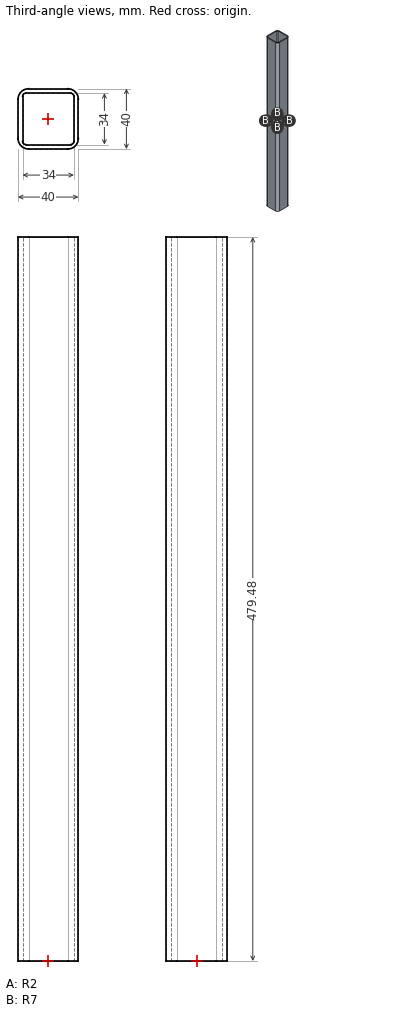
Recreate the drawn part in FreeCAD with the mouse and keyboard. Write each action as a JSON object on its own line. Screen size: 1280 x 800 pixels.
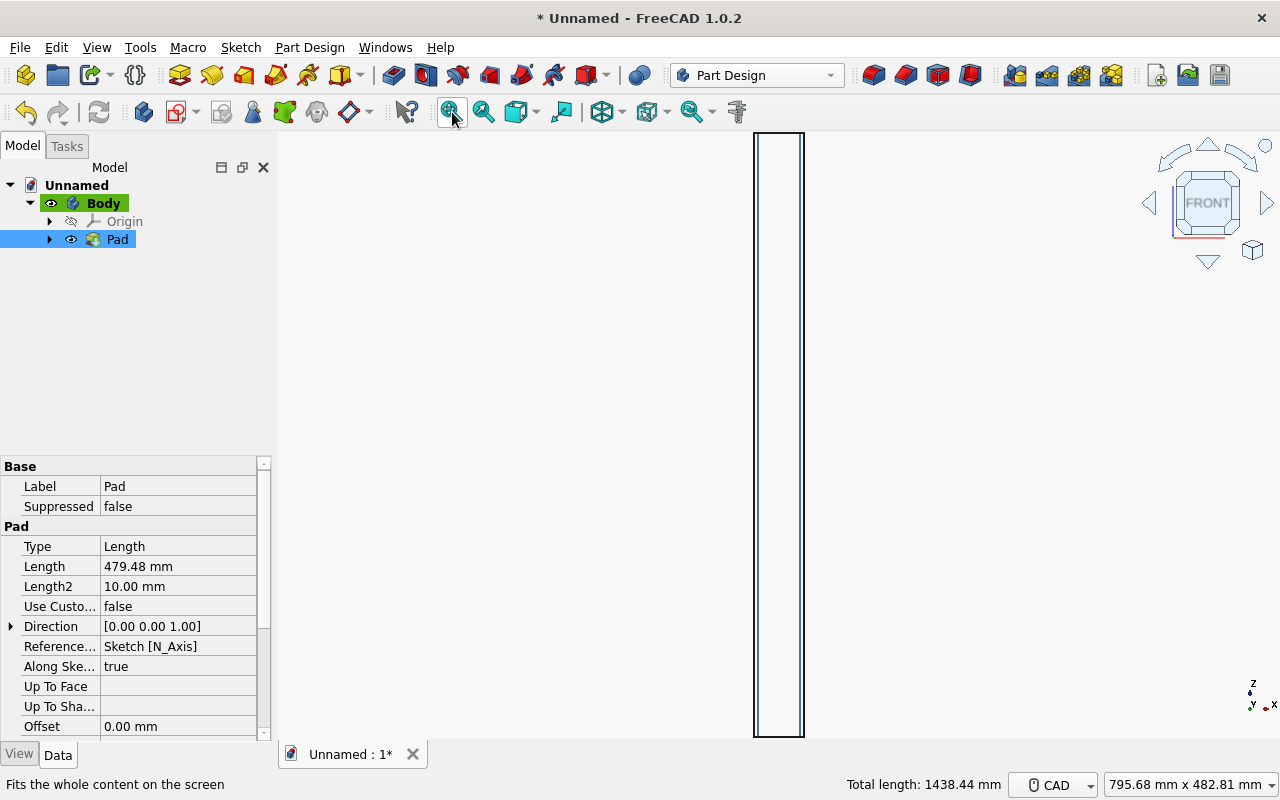
{"action": "key", "text": "3"}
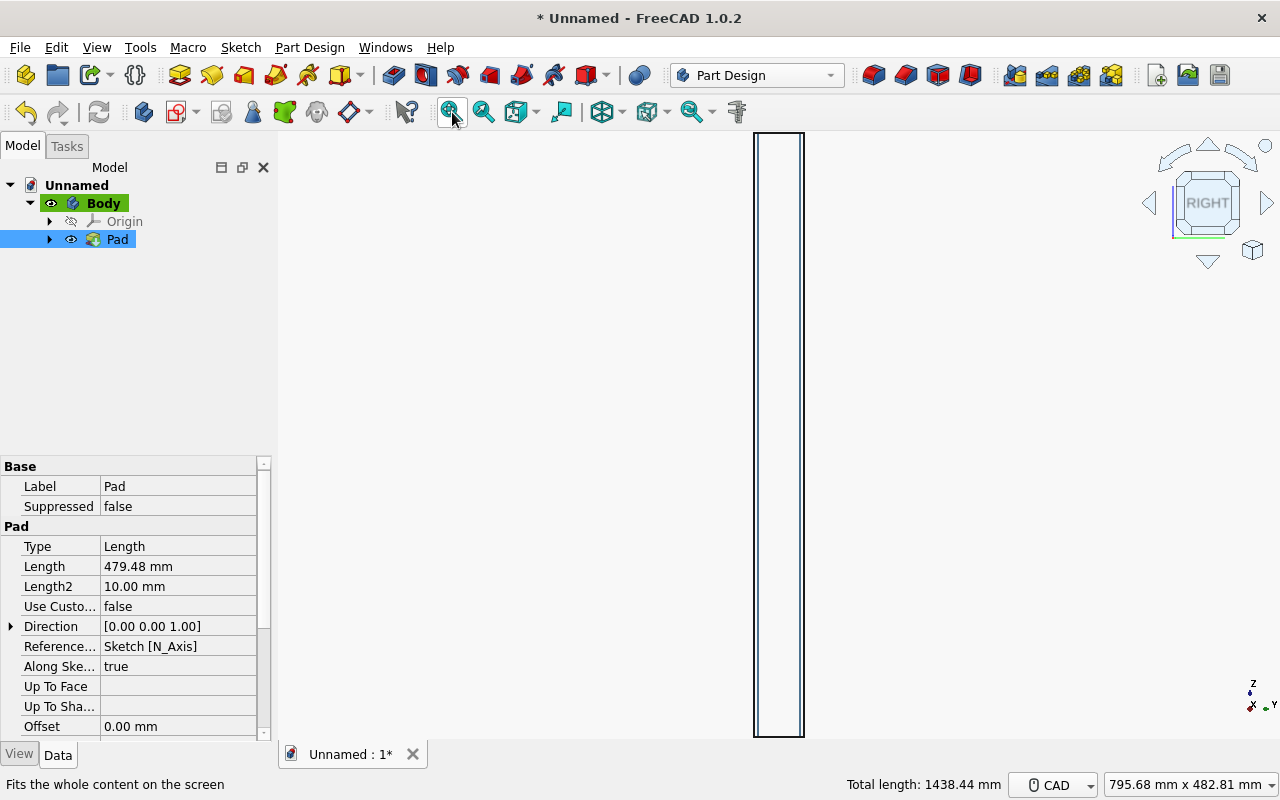
{"action": "scroll", "coordinate": [800, 434], "scroll_direction": "up", "scroll_amount": 6}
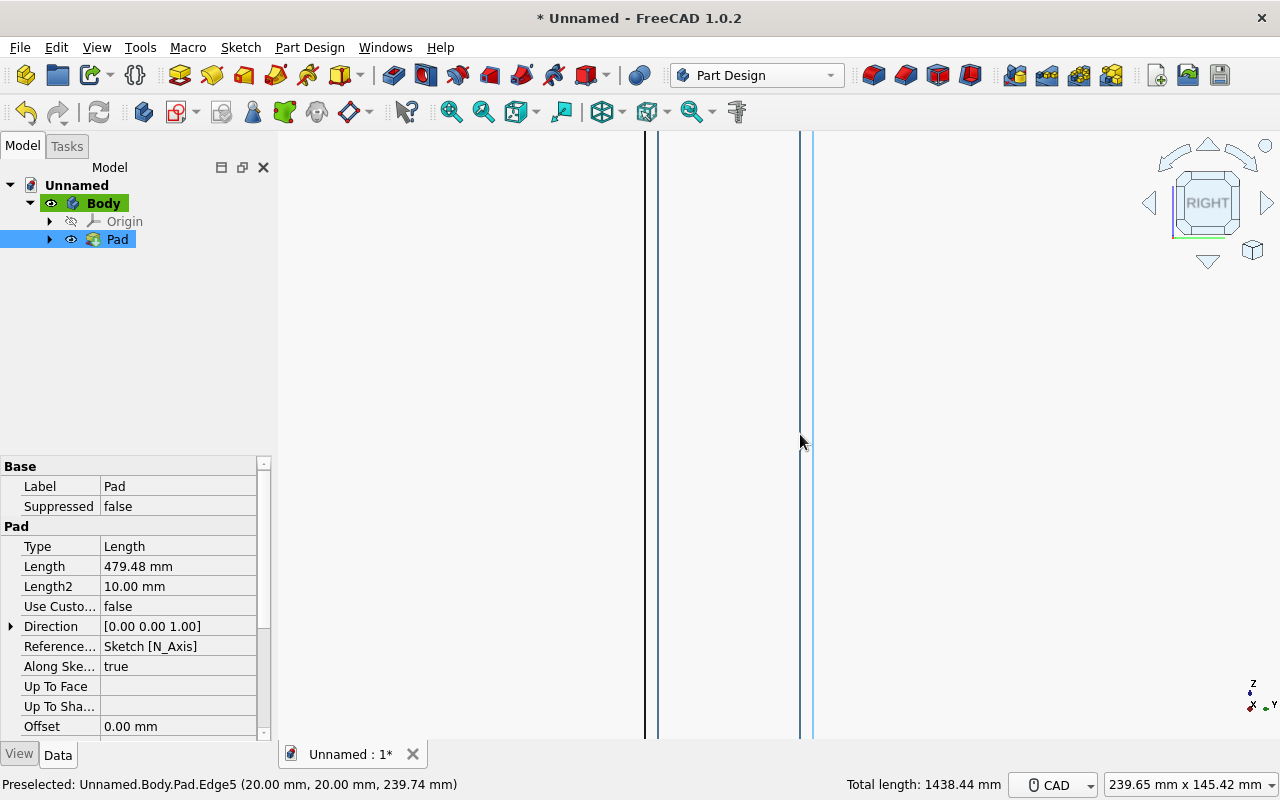
{"action": "key", "text": "v f"}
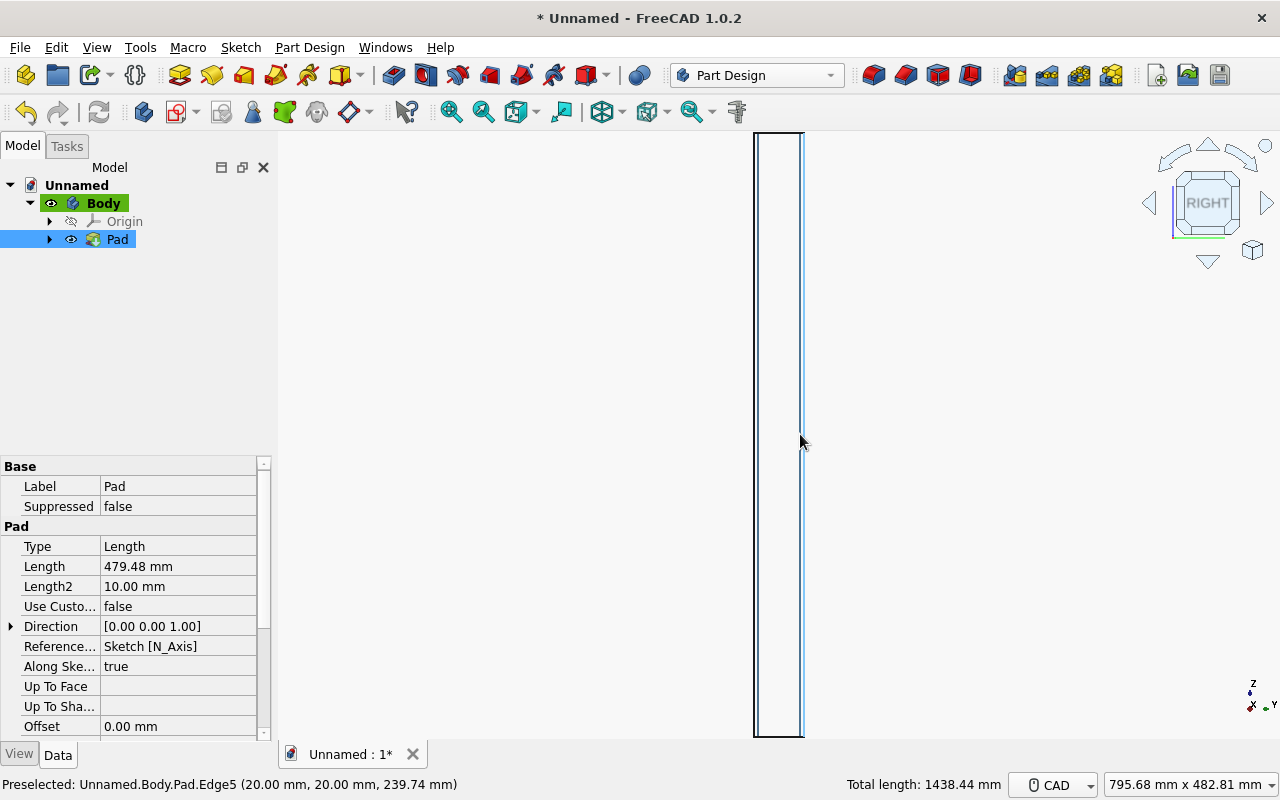
{"action": "key", "text": "5"}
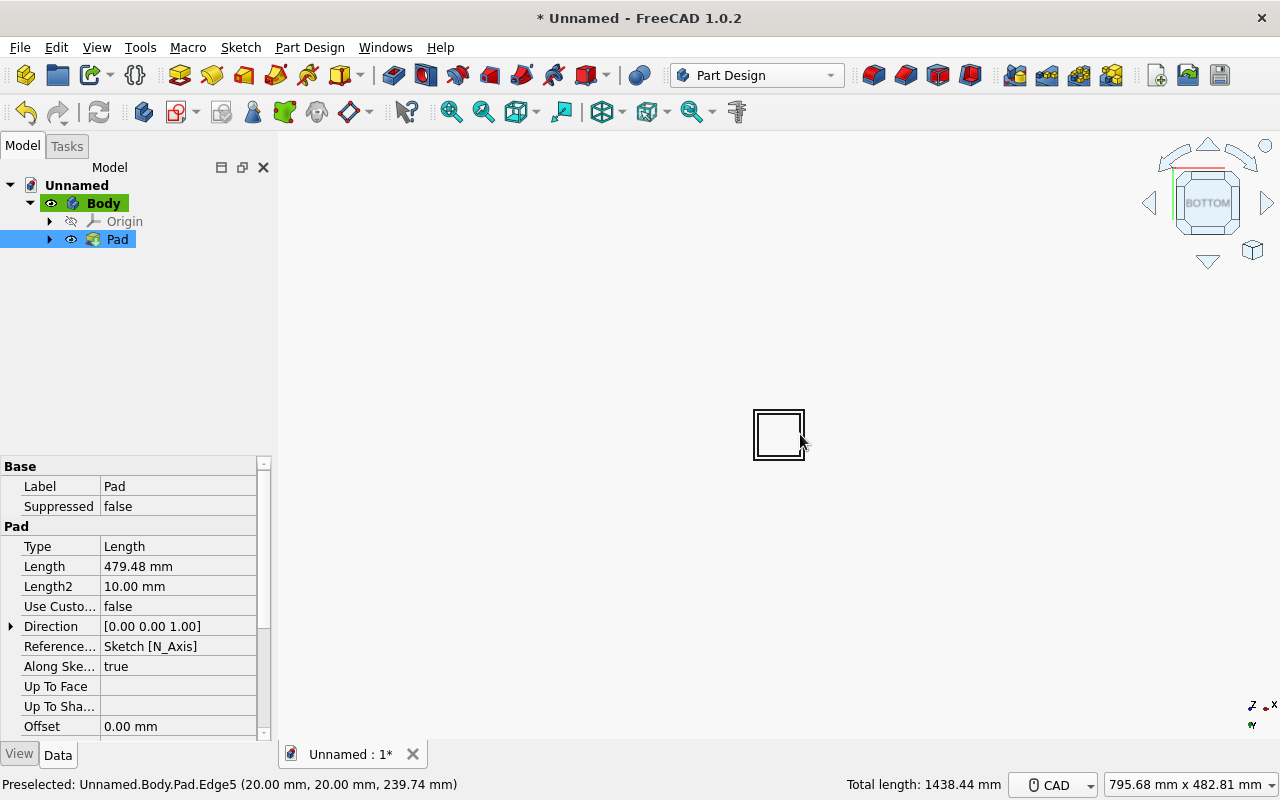
{"action": "key", "text": "v f"}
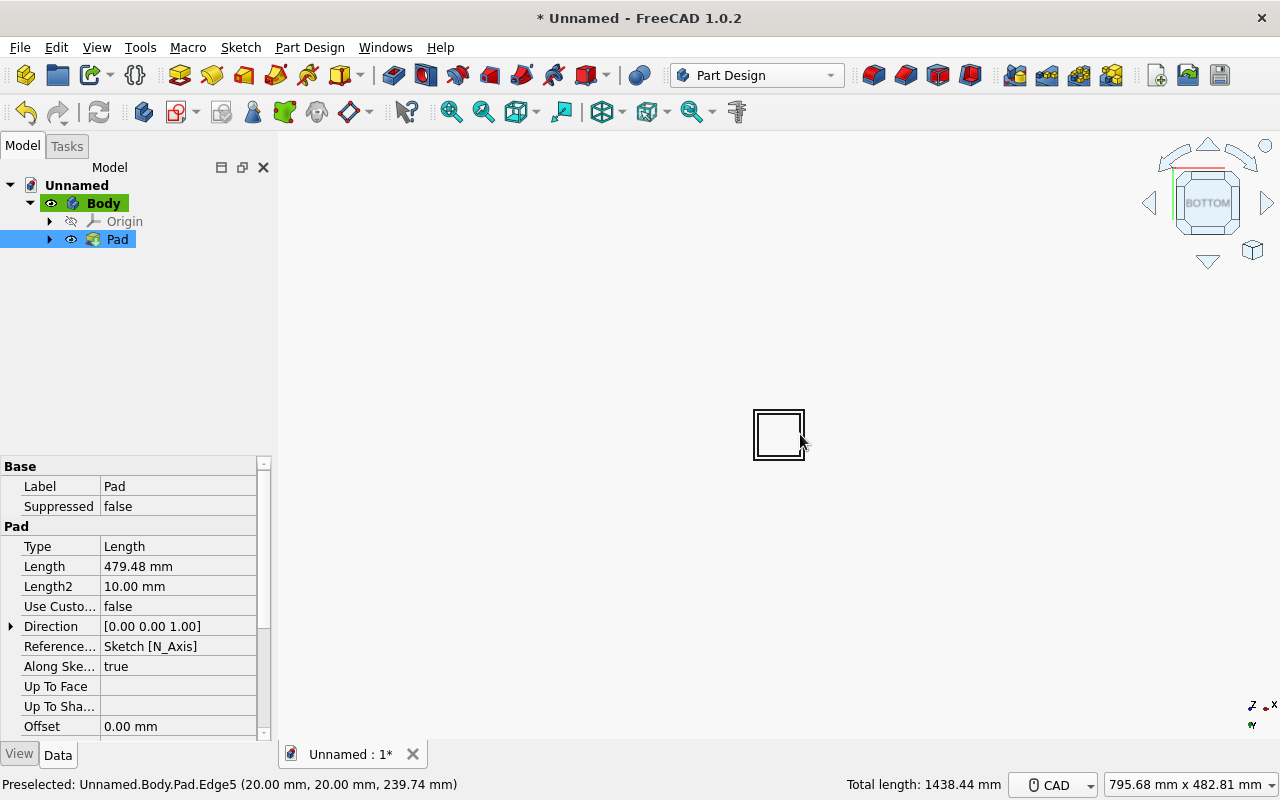
{"action": "scroll", "coordinate": [758, 455], "scroll_direction": "up", "scroll_amount": 6}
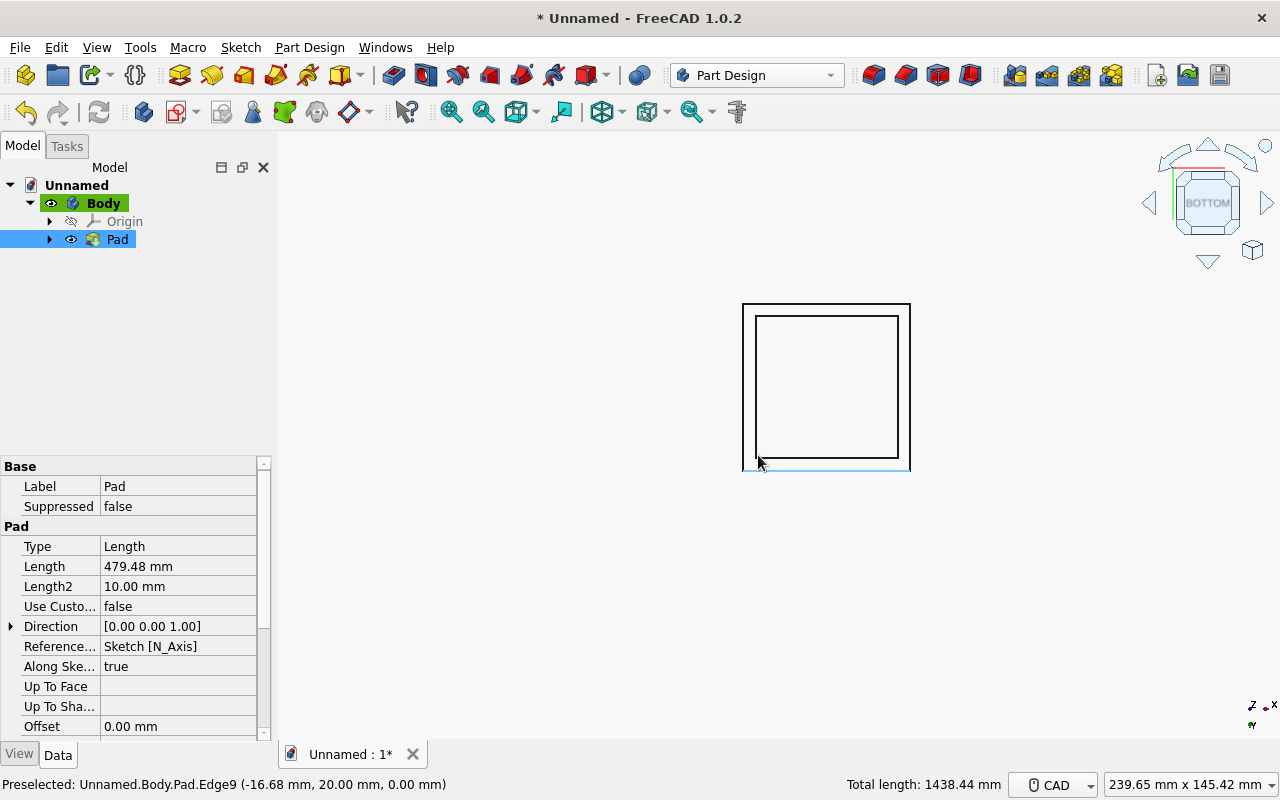
{"action": "key", "text": "v f"}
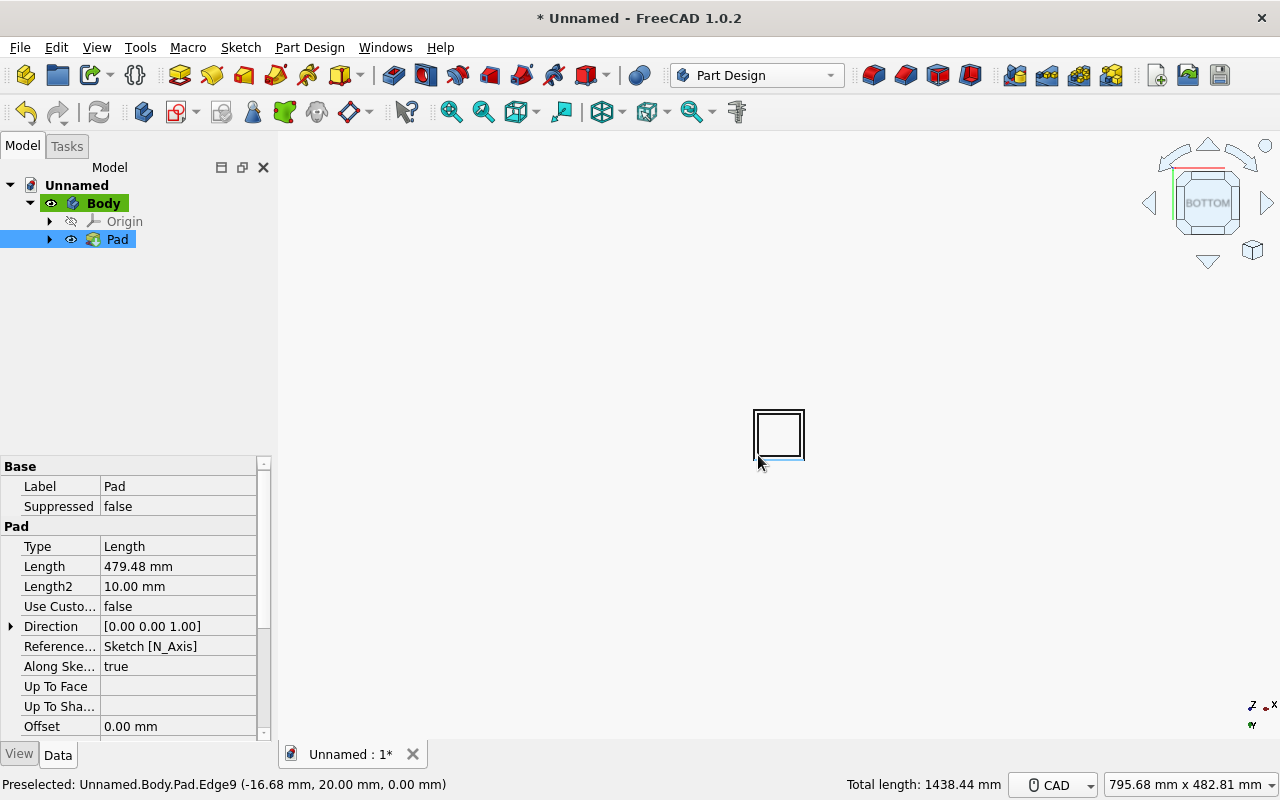
{"action": "key", "text": "4"}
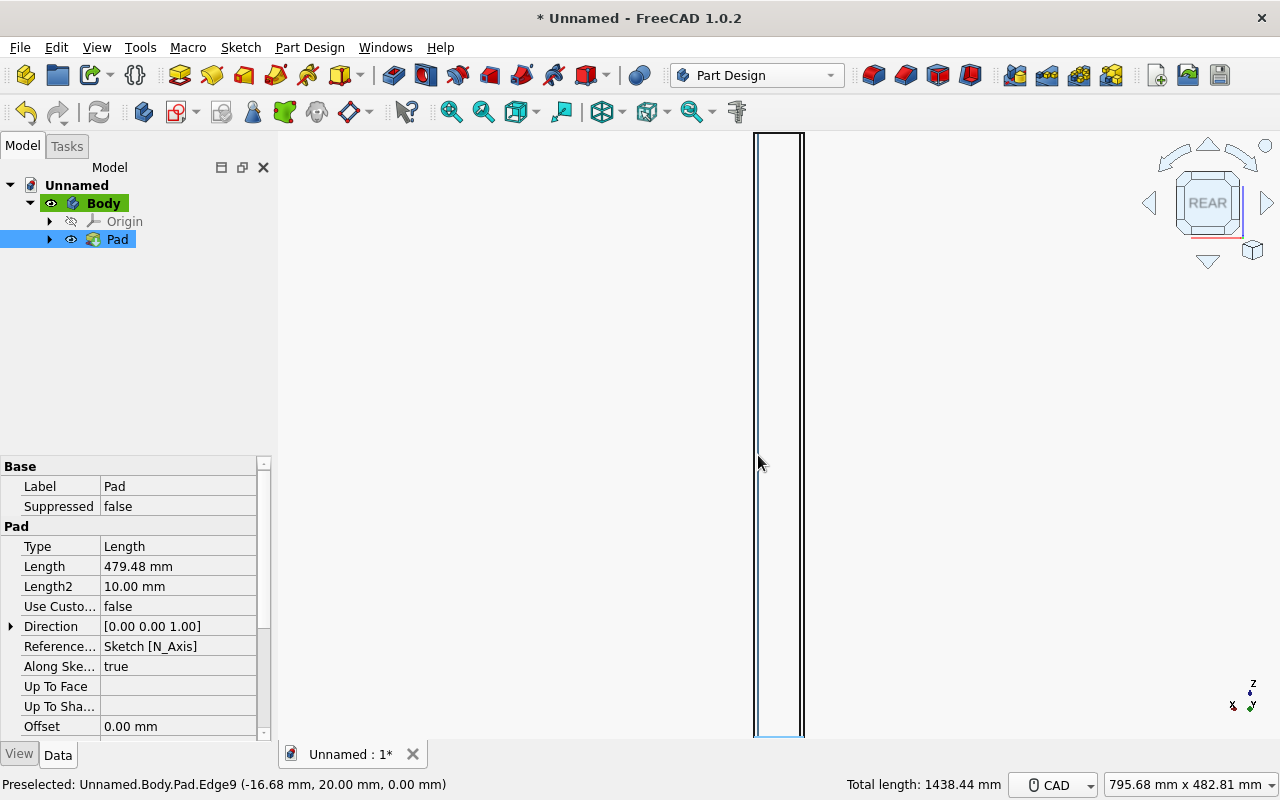
{"action": "scroll", "coordinate": [800, 434], "scroll_direction": "up", "scroll_amount": 6}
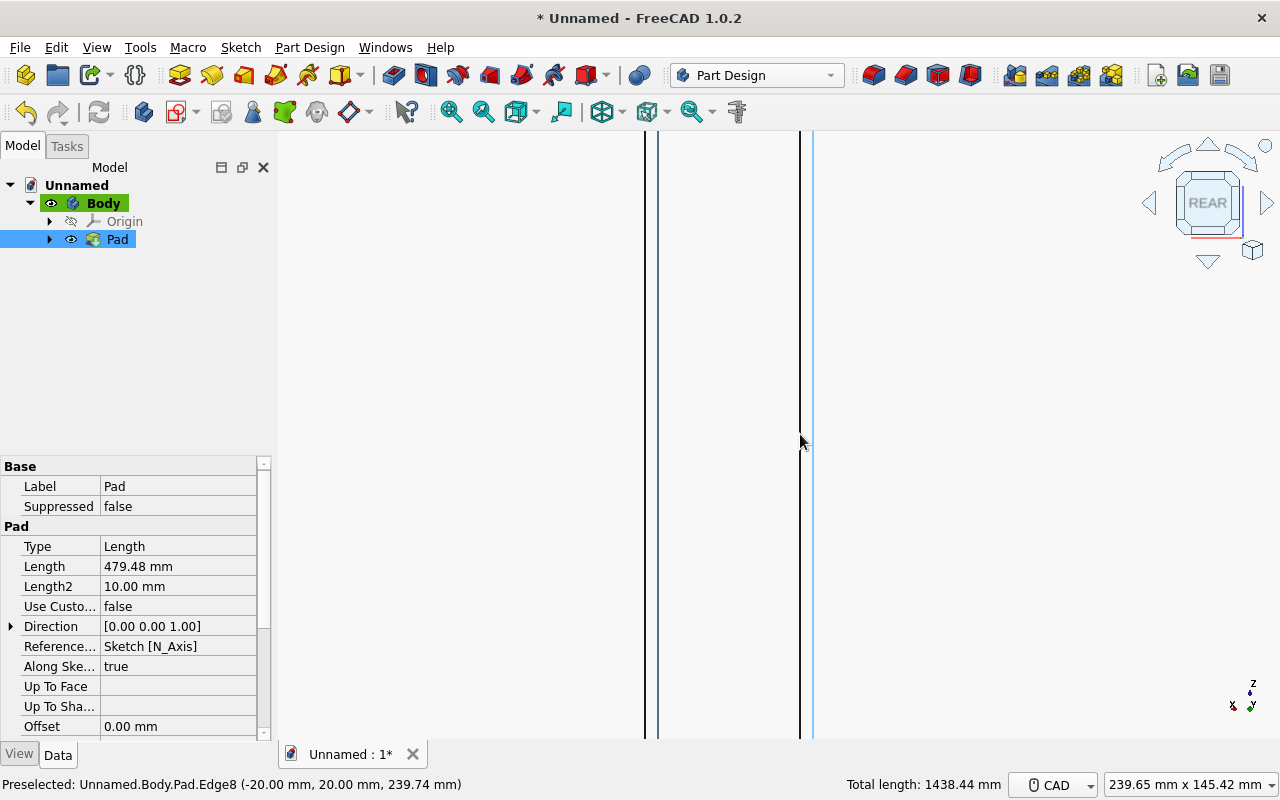
{"action": "left_click", "coordinate": [800, 435], "text": "ctrl"}